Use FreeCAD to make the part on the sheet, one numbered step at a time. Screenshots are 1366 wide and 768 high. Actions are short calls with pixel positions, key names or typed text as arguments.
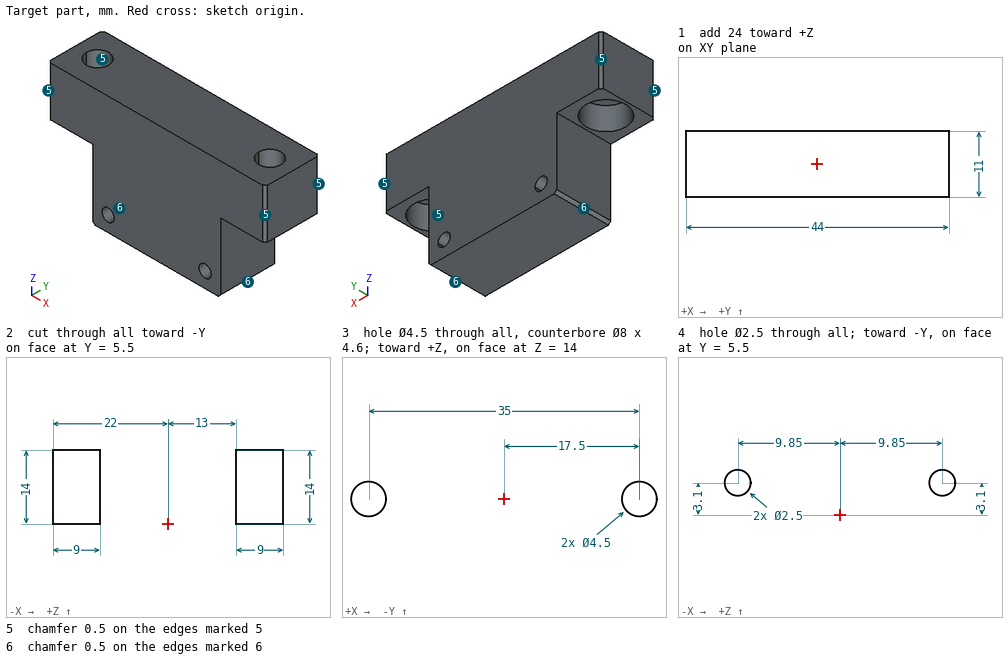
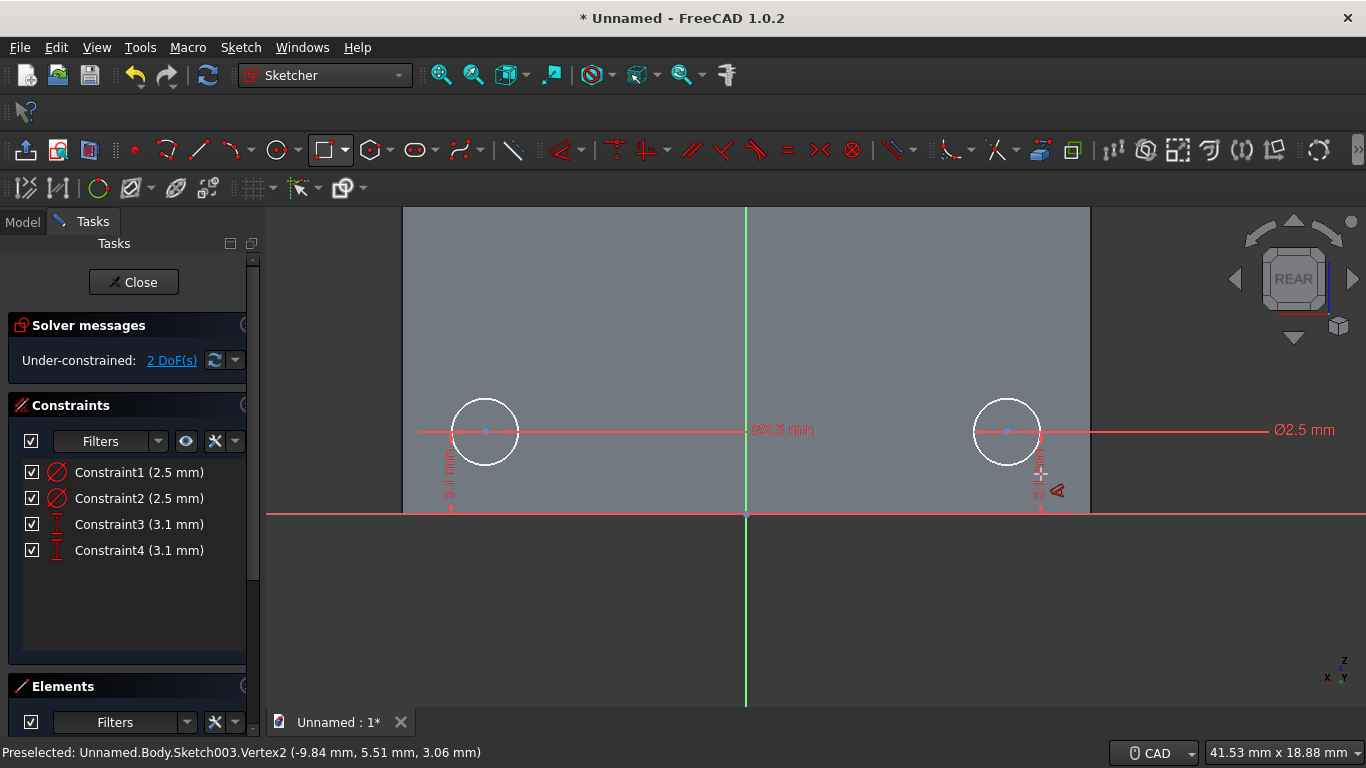
click(485, 432)
click(616, 548)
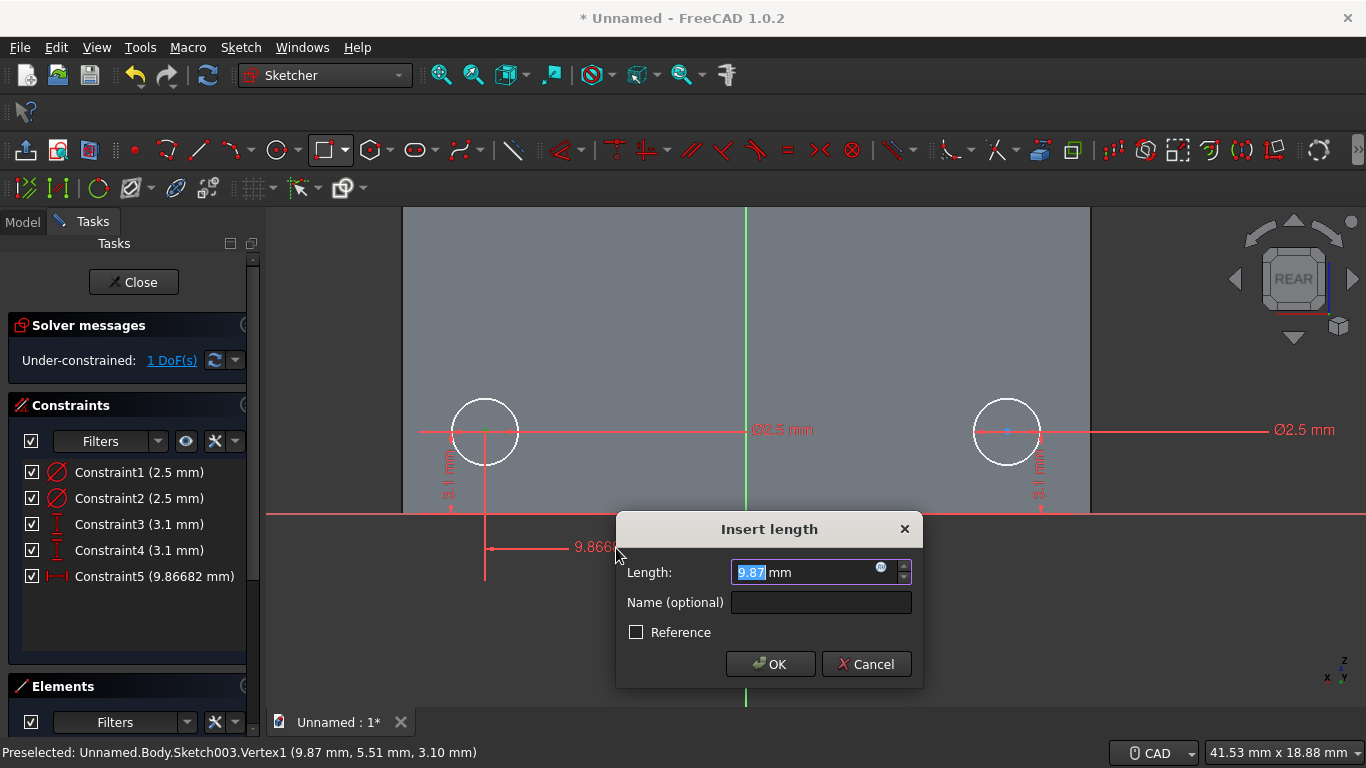
text(9.85)
key(Return)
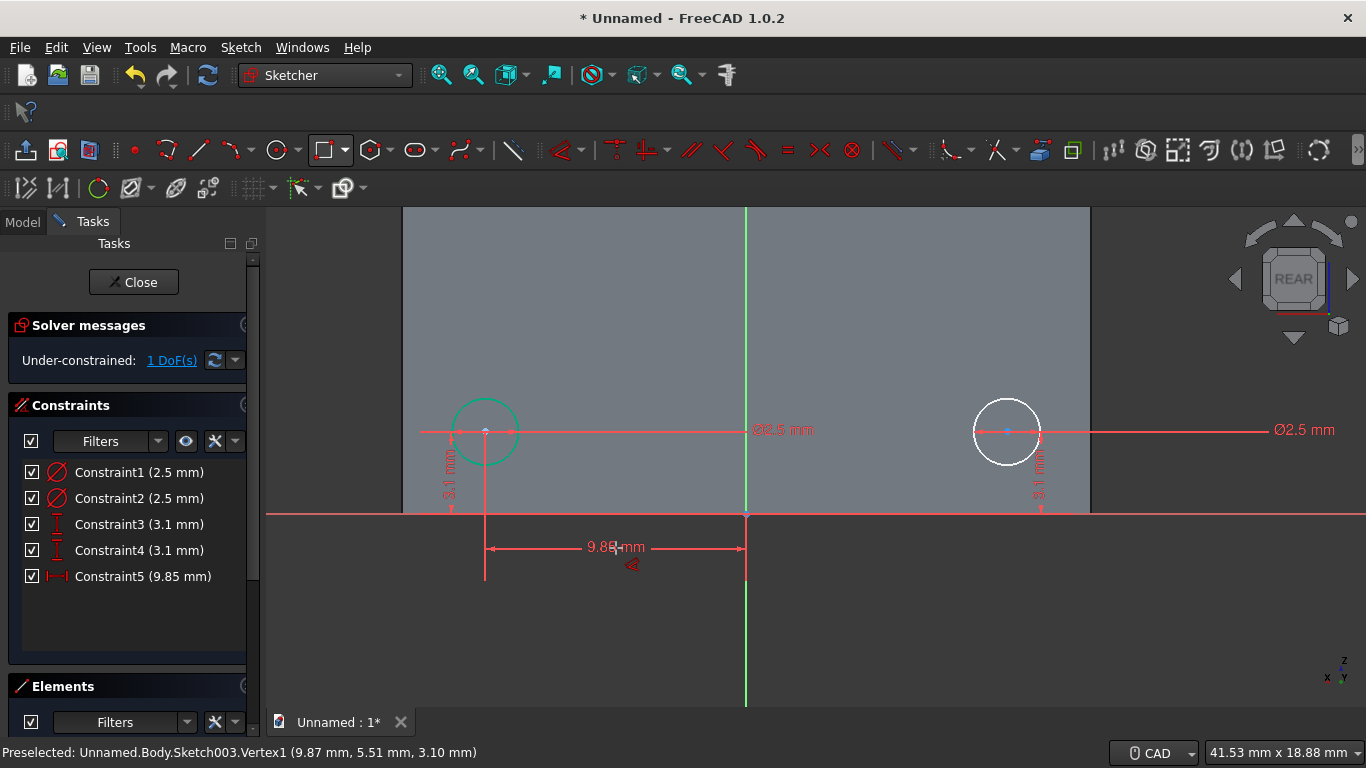
click(1007, 432)
click(877, 548)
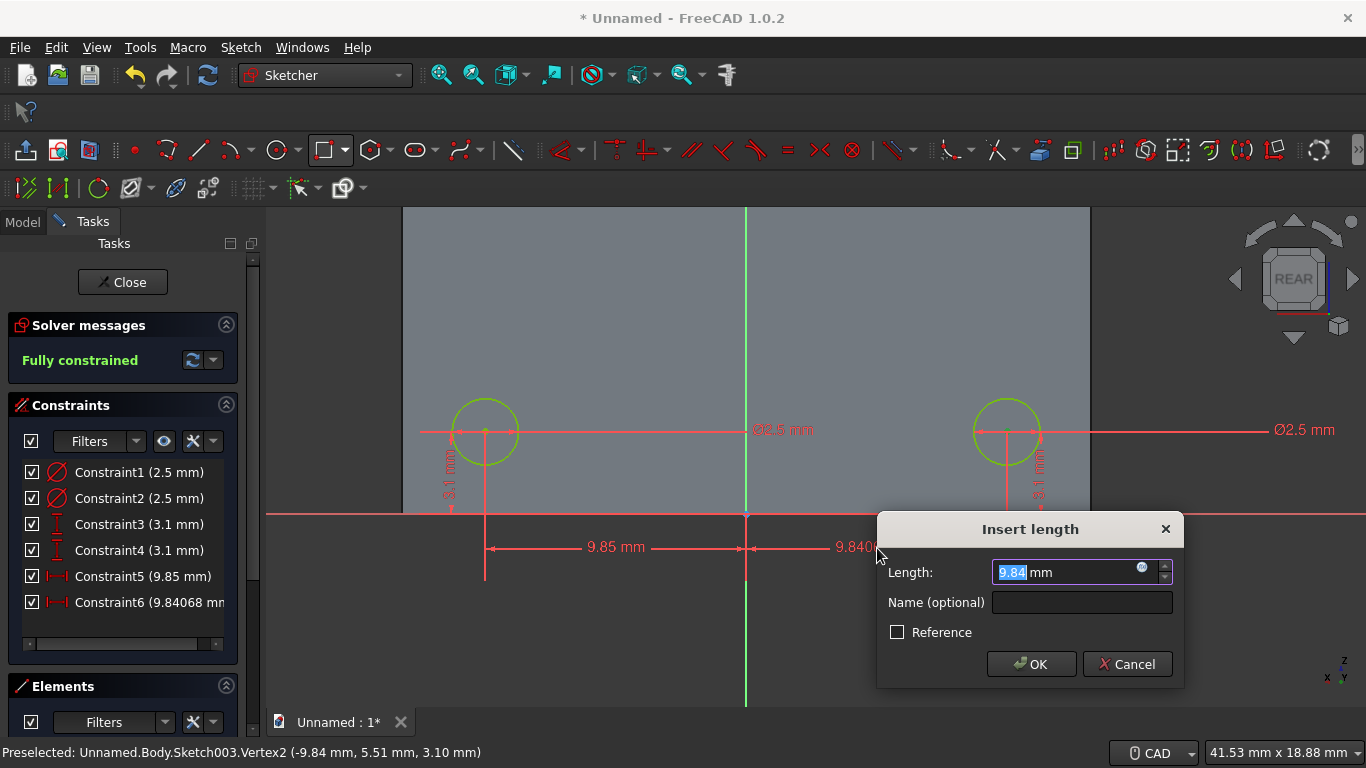
text(9.85)
key(Return)
key(Escape)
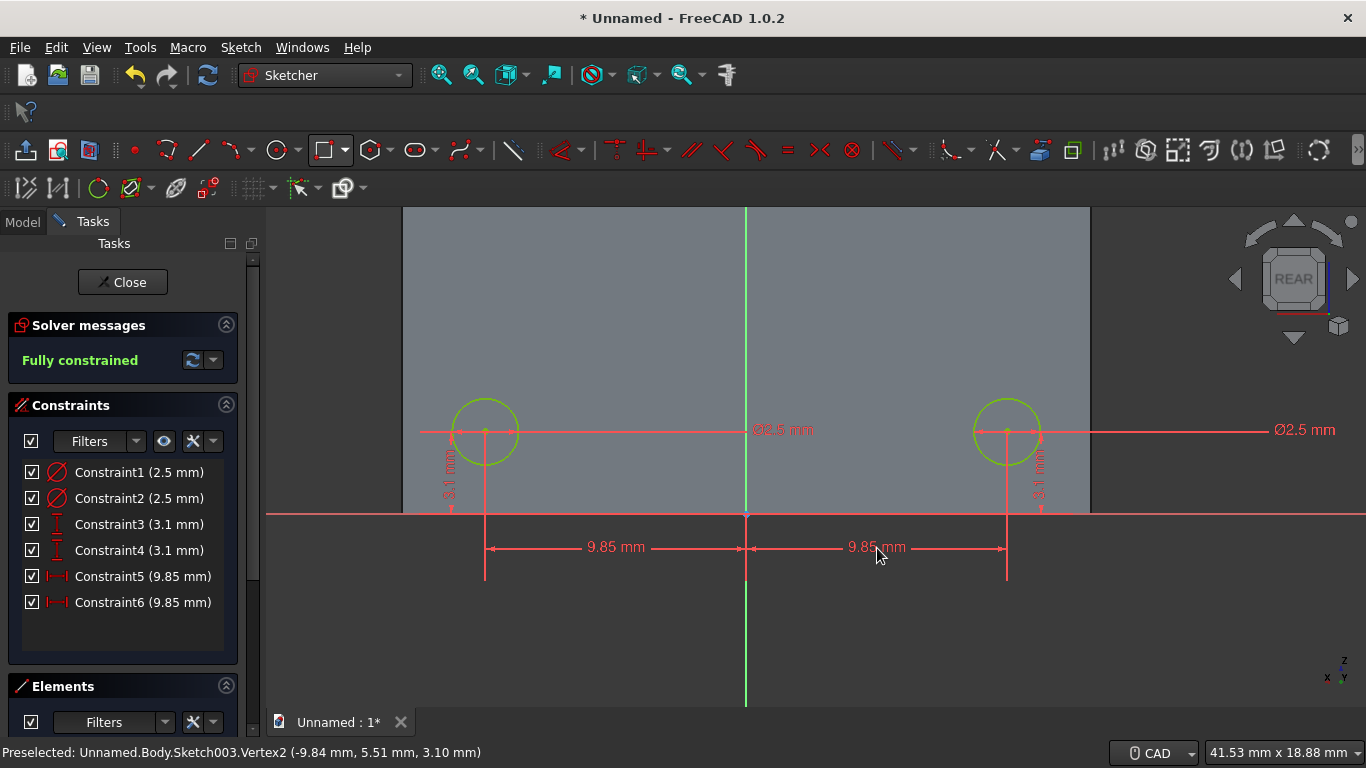
click(123, 282)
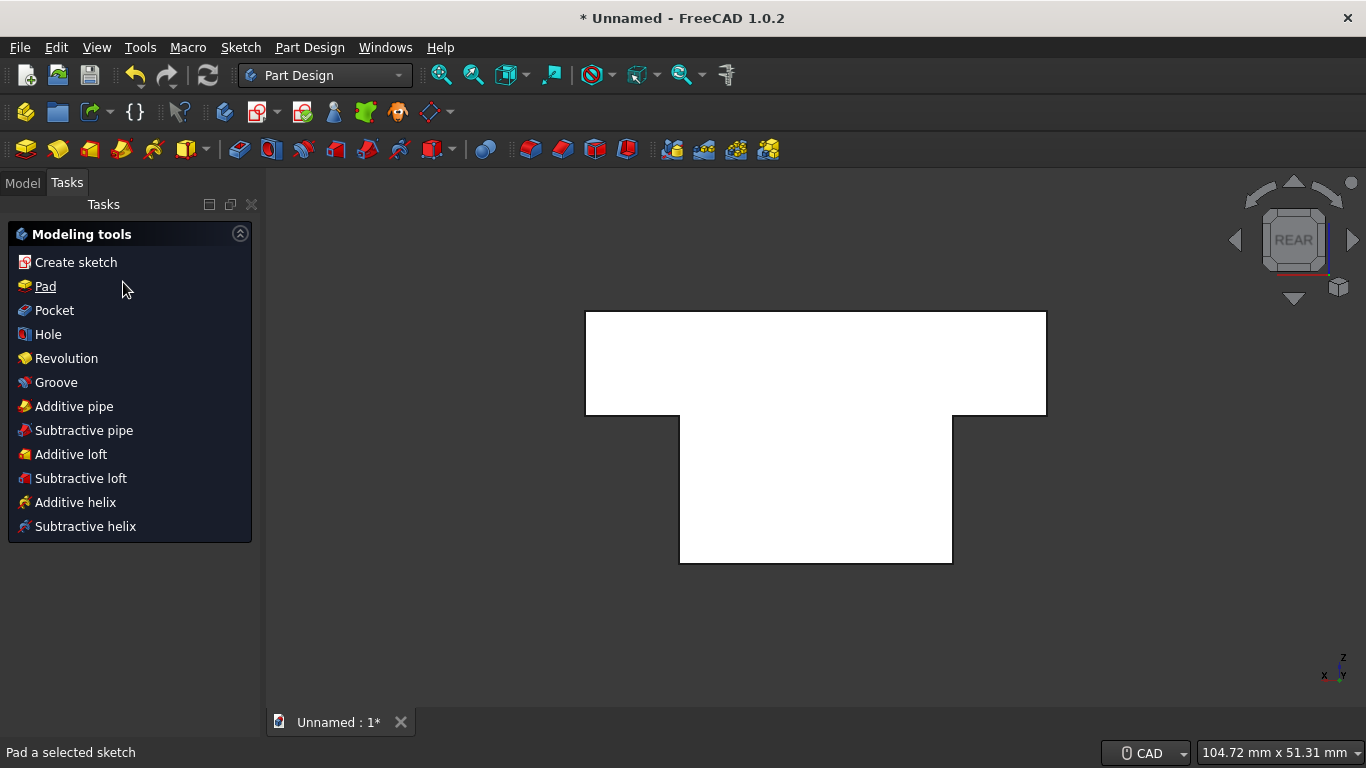
click(272, 150)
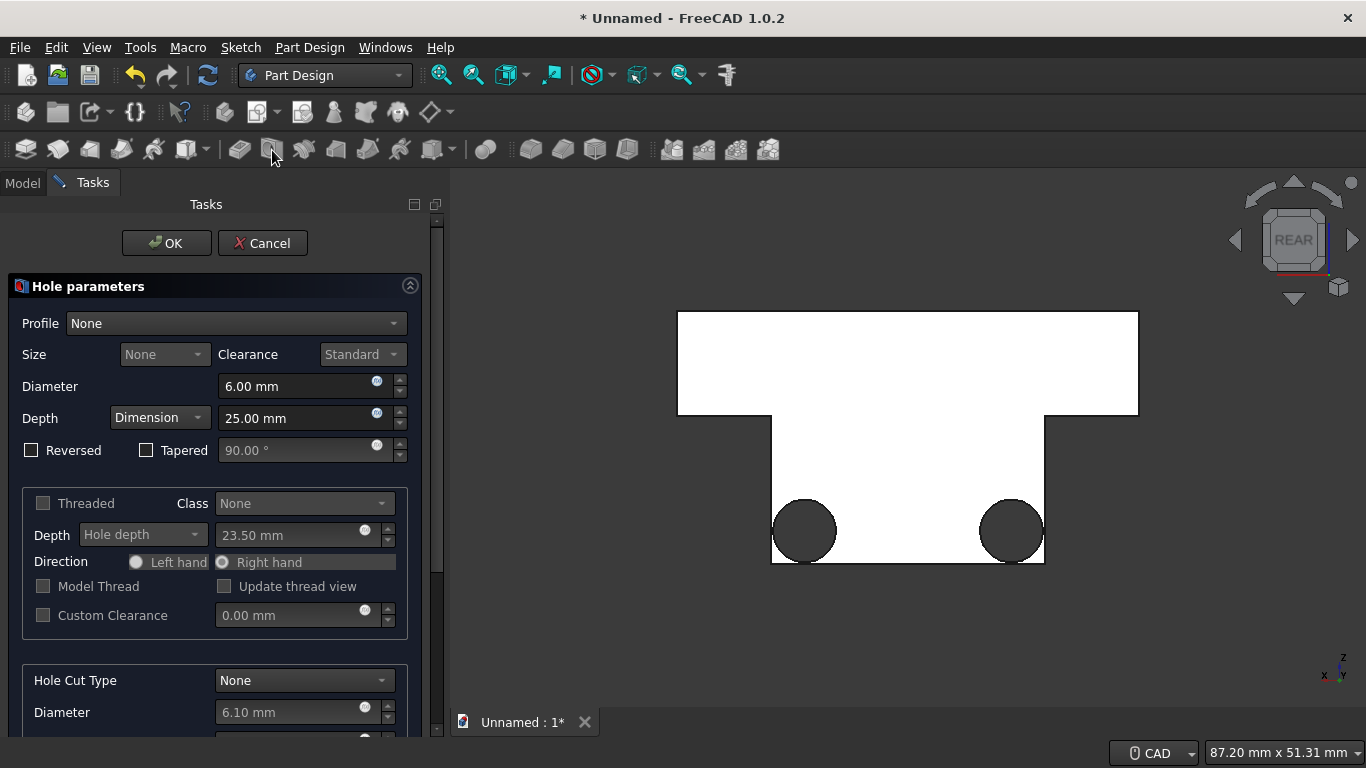
triple_click(305, 386)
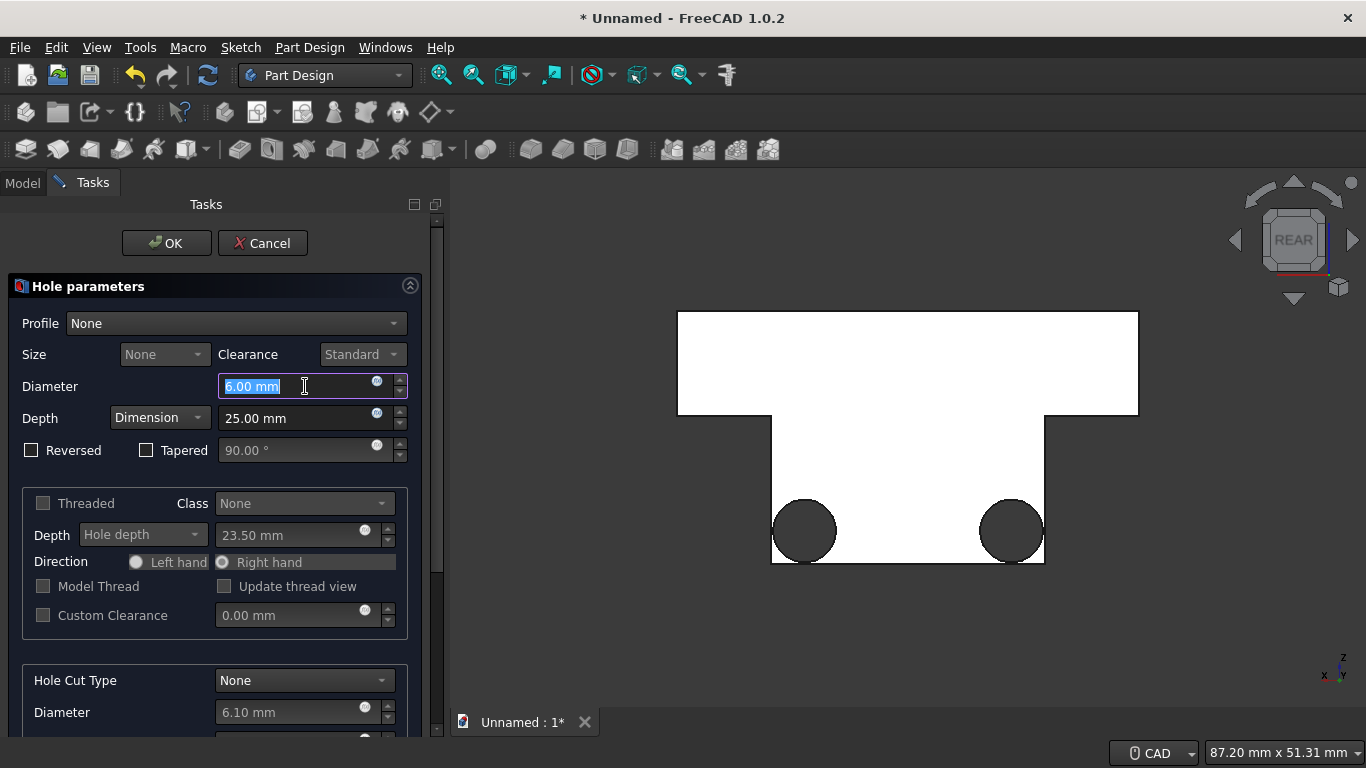
text(2.5)
key(Tab)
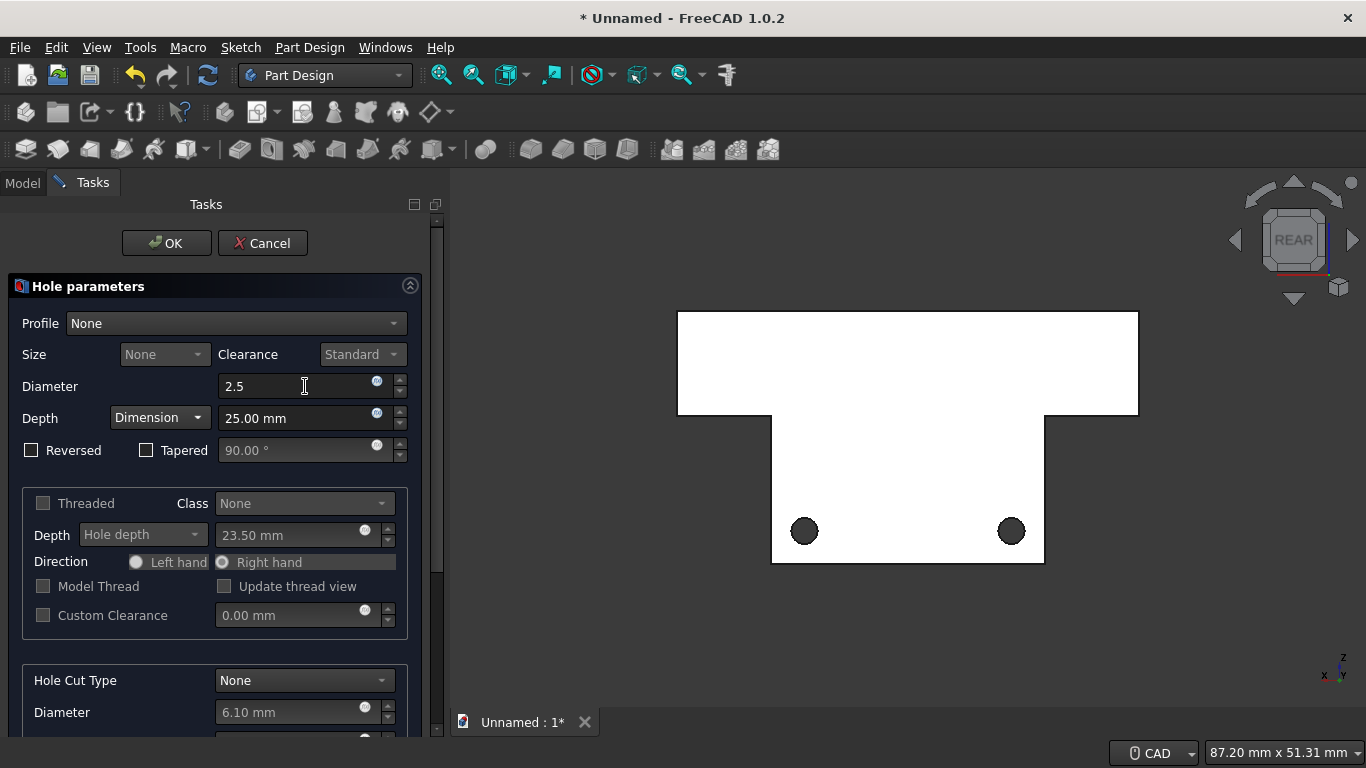
click(161, 418)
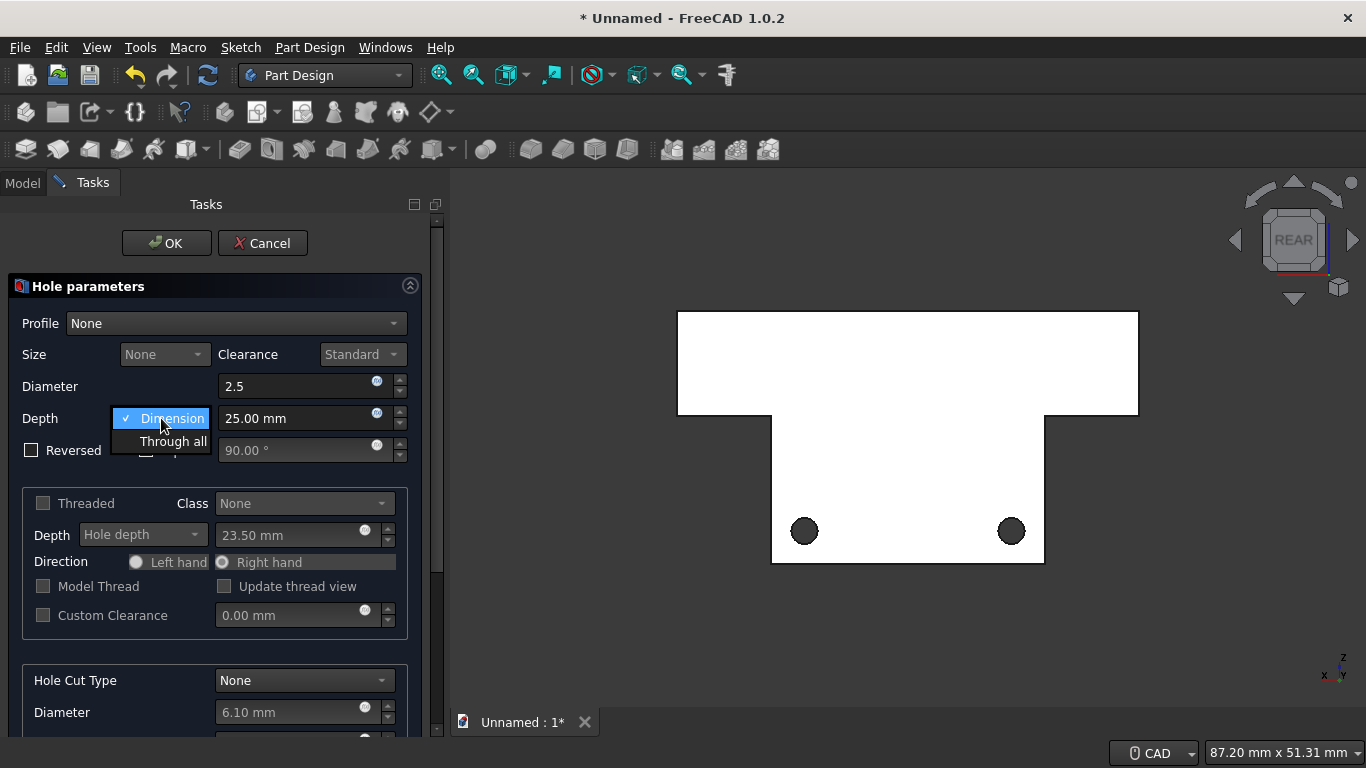
click(160, 442)